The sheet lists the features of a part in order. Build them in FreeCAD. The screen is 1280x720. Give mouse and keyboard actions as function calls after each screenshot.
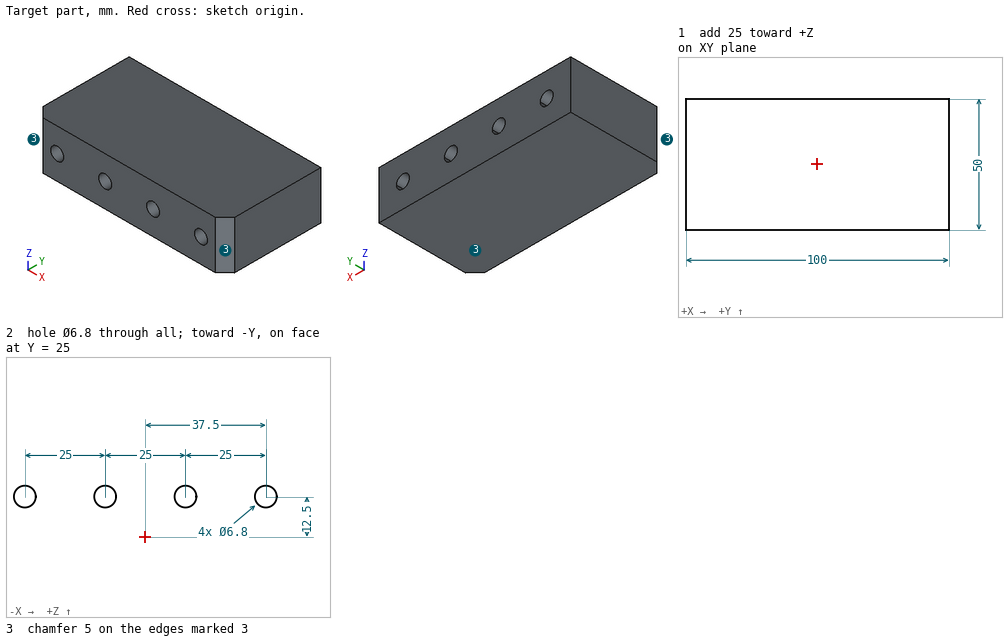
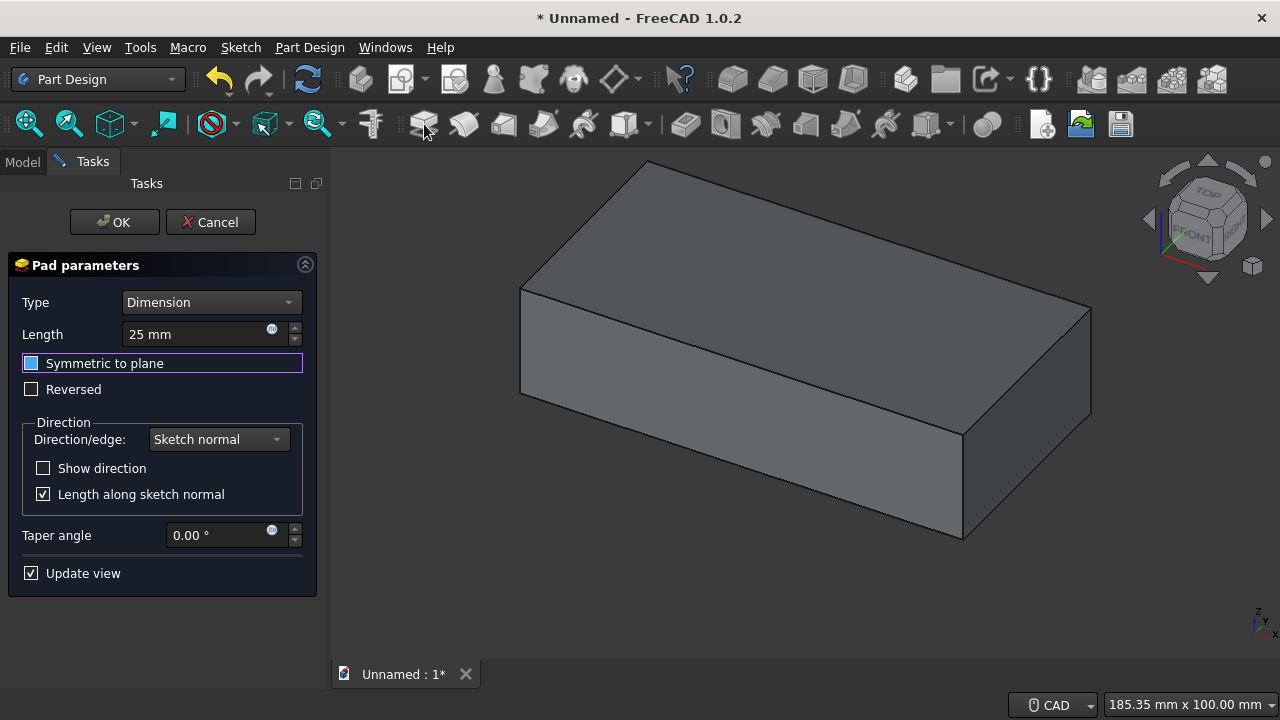
click(115, 222)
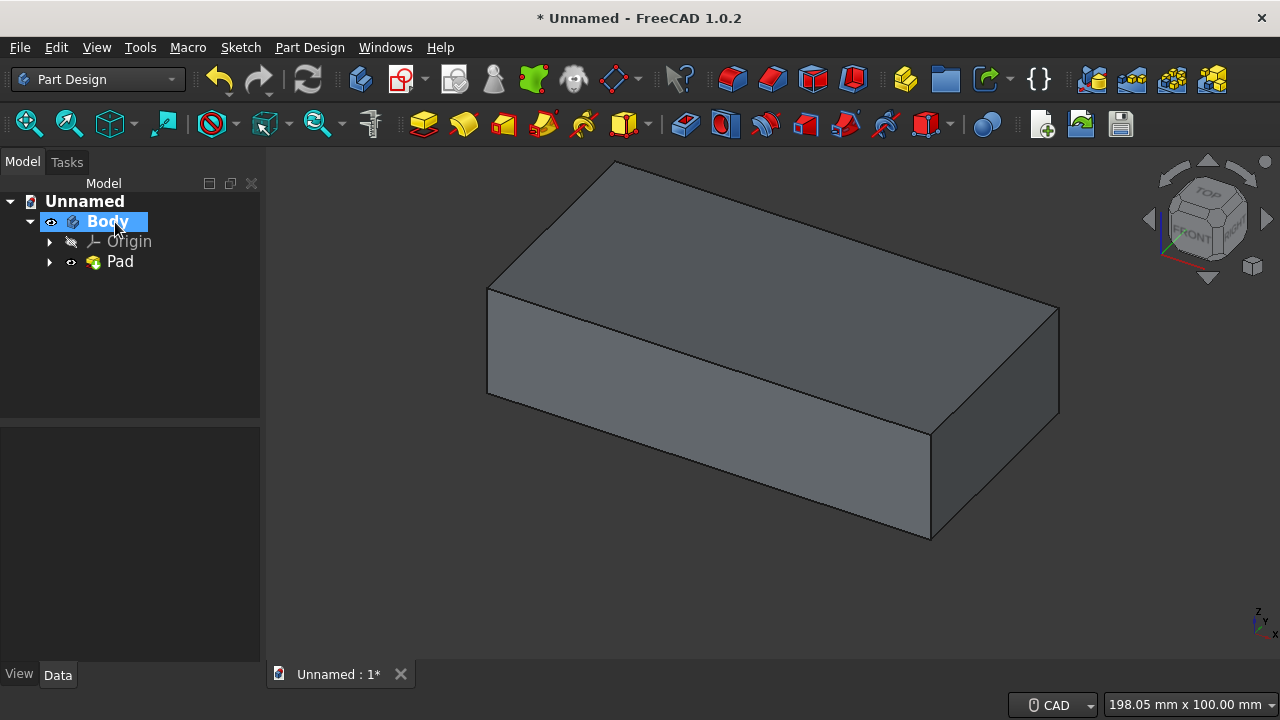
key(4)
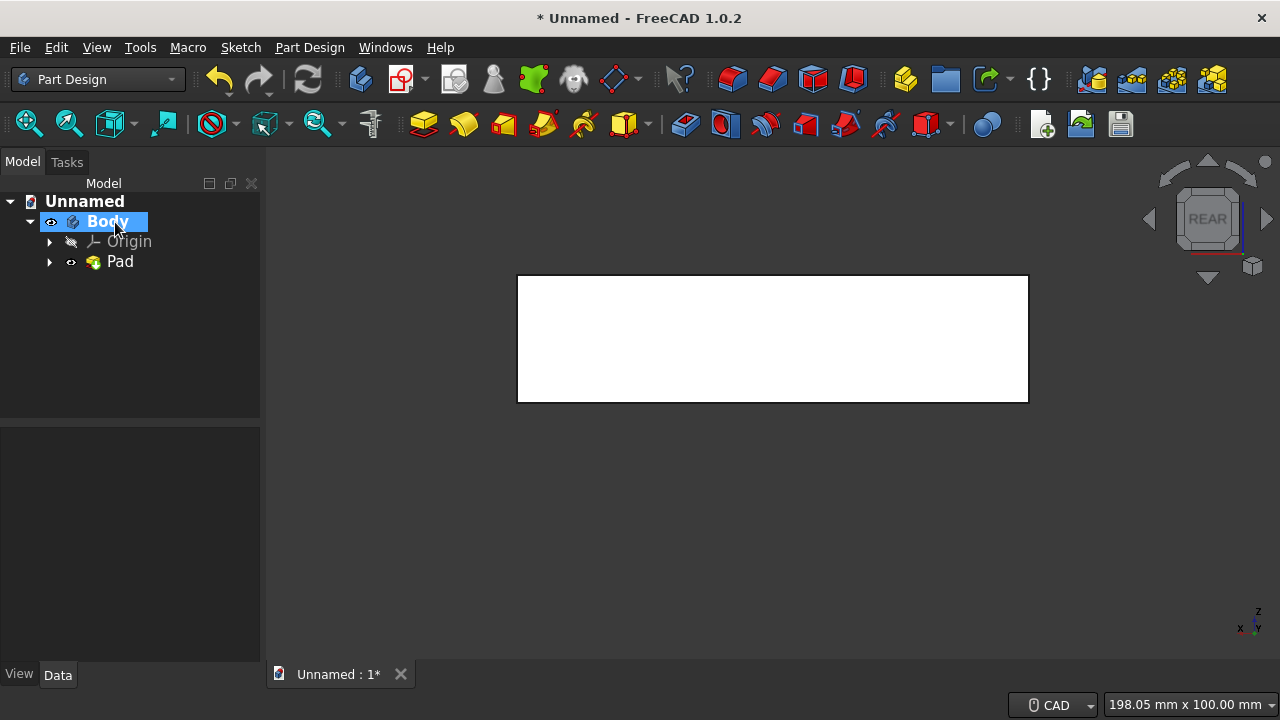
click(627, 338)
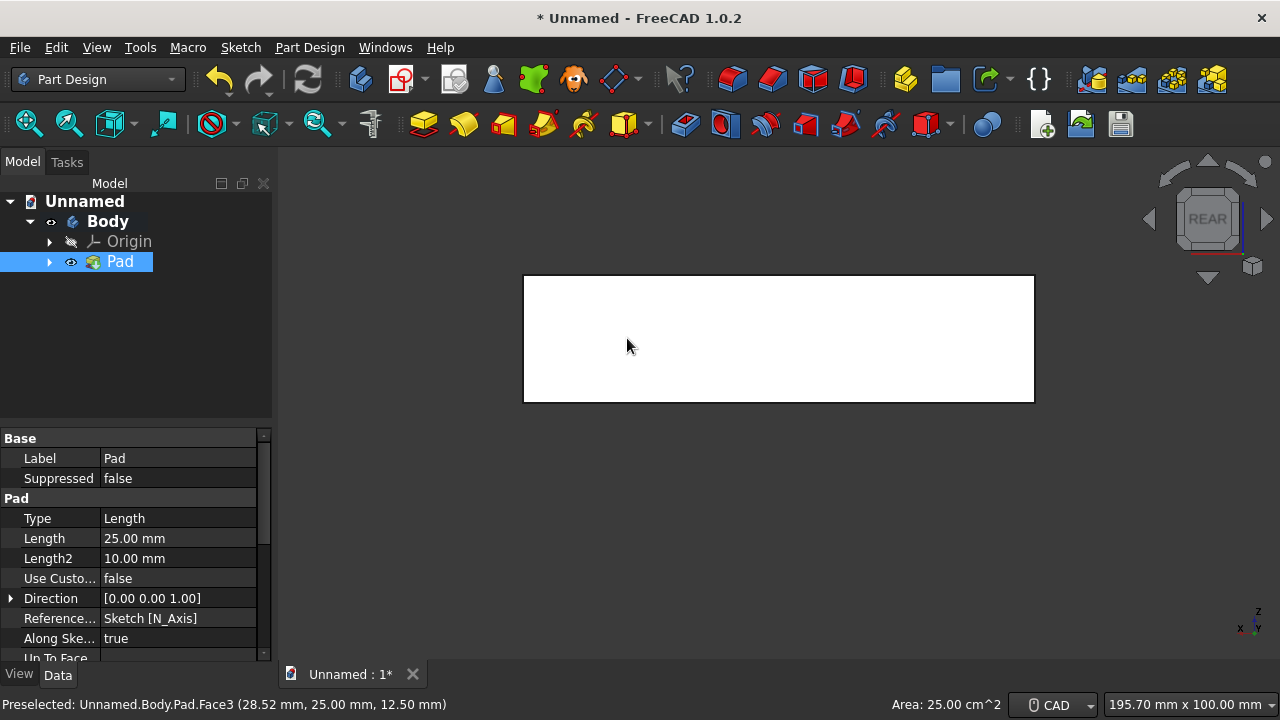
click(402, 80)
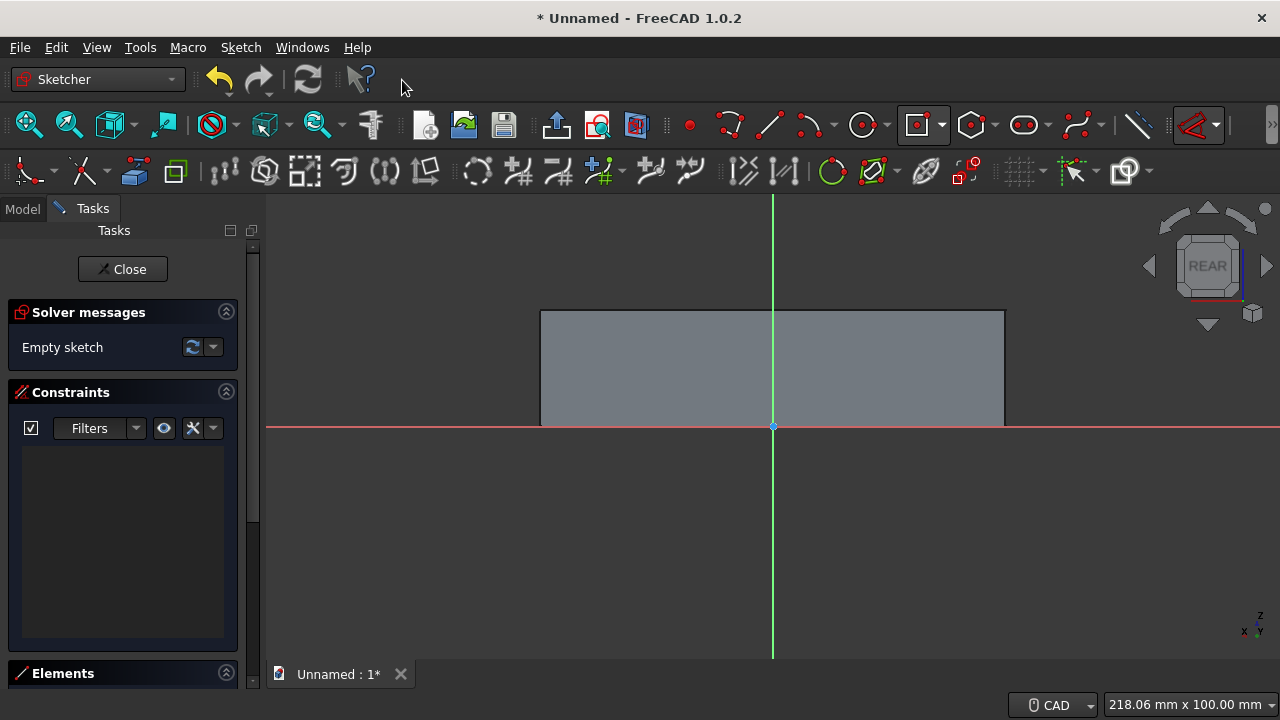
scroll(912, 314, up, 2)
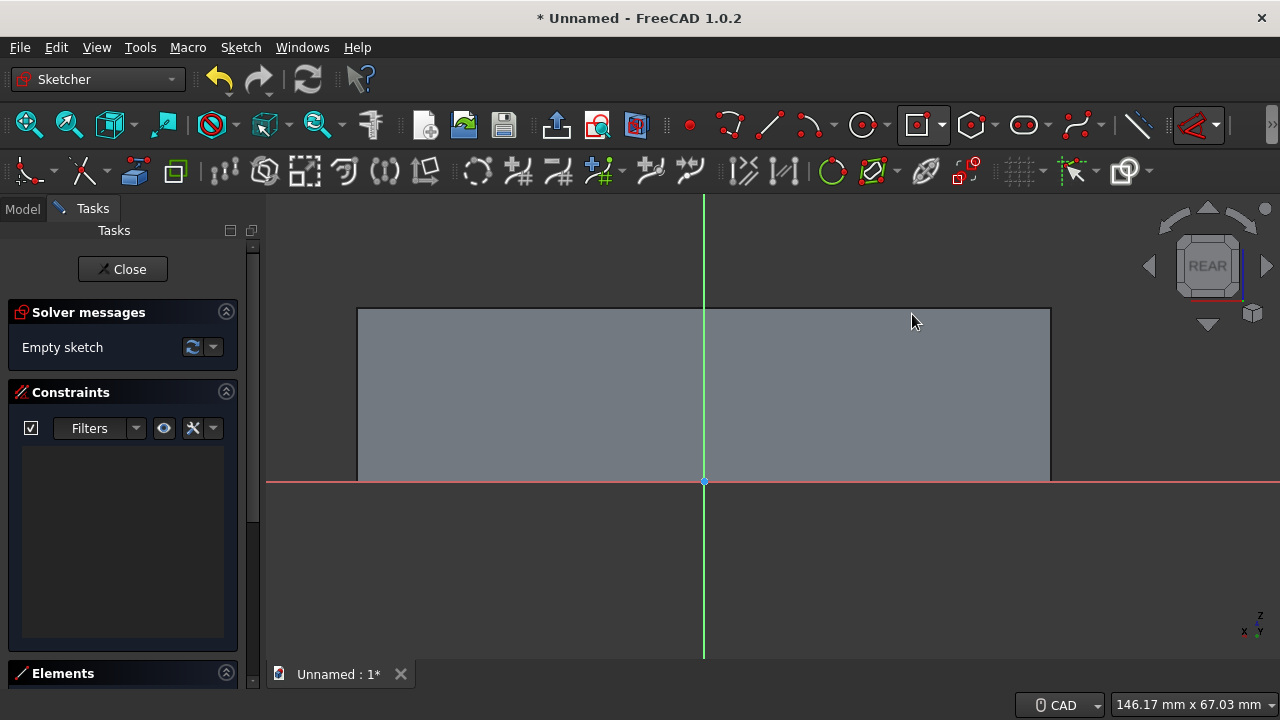
click(864, 126)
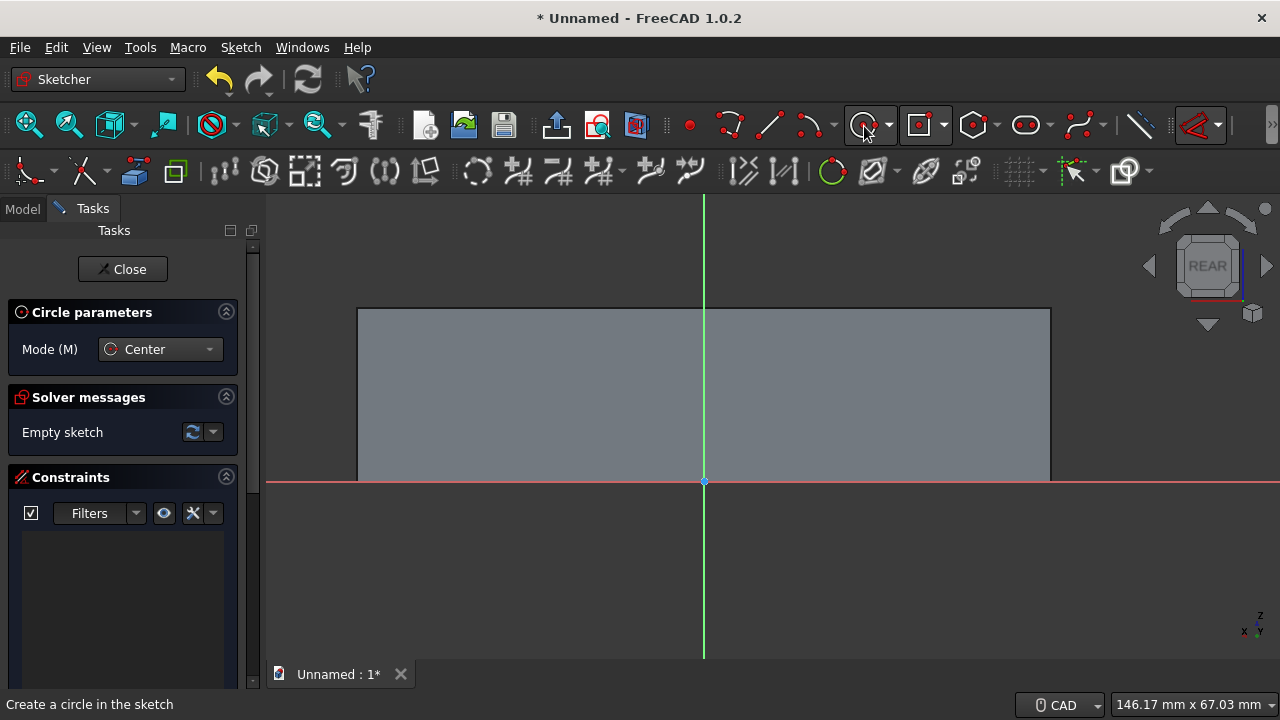
click(964, 395)
move(981, 378)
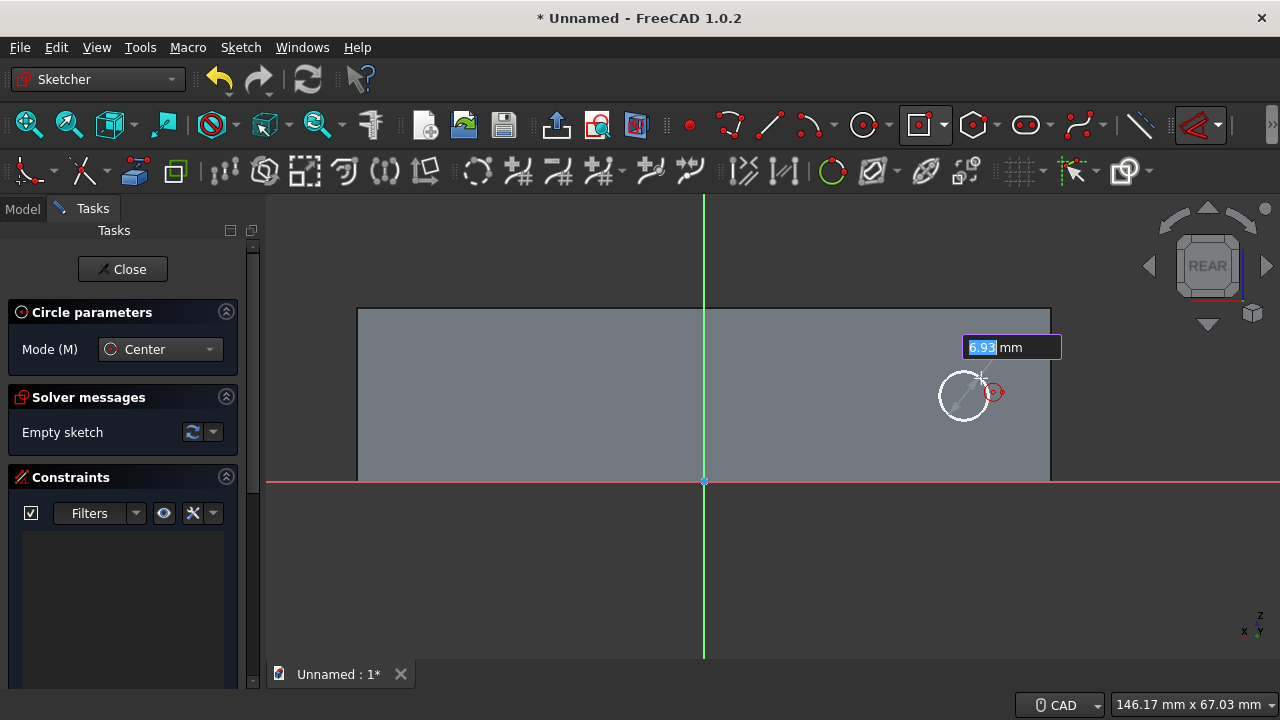
text(6.8)
key(Return)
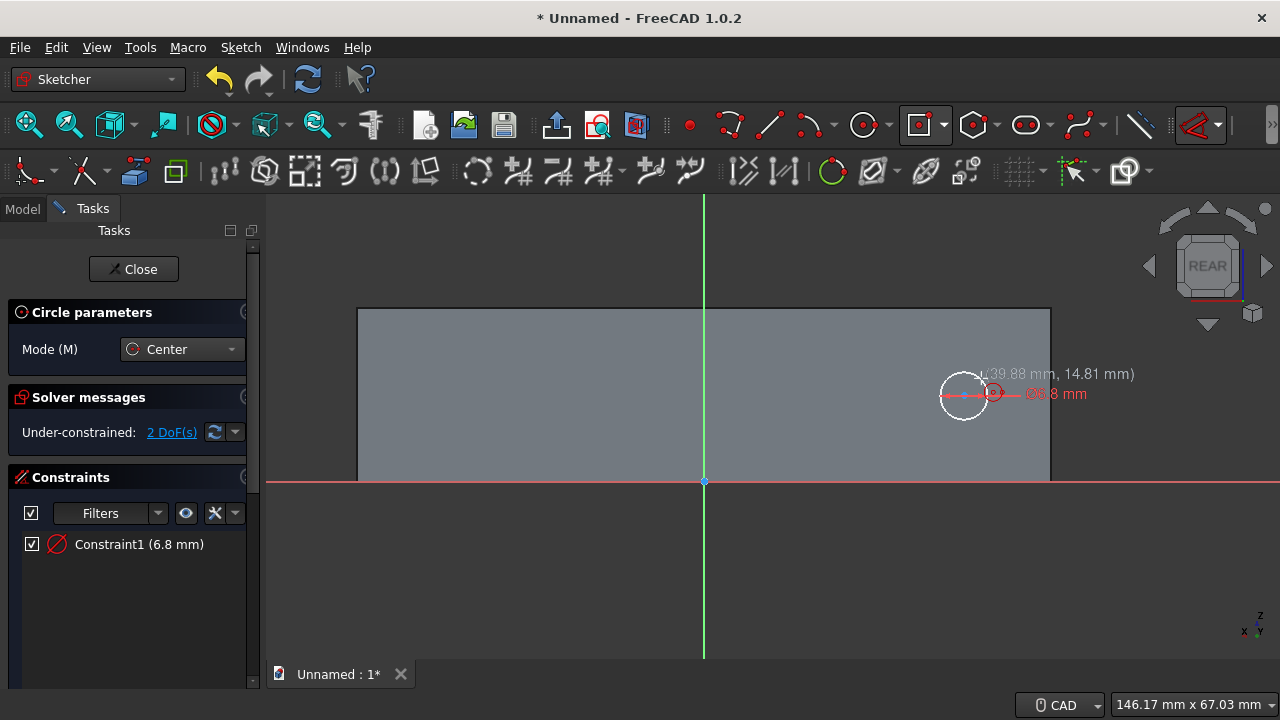
click(791, 395)
move(808, 378)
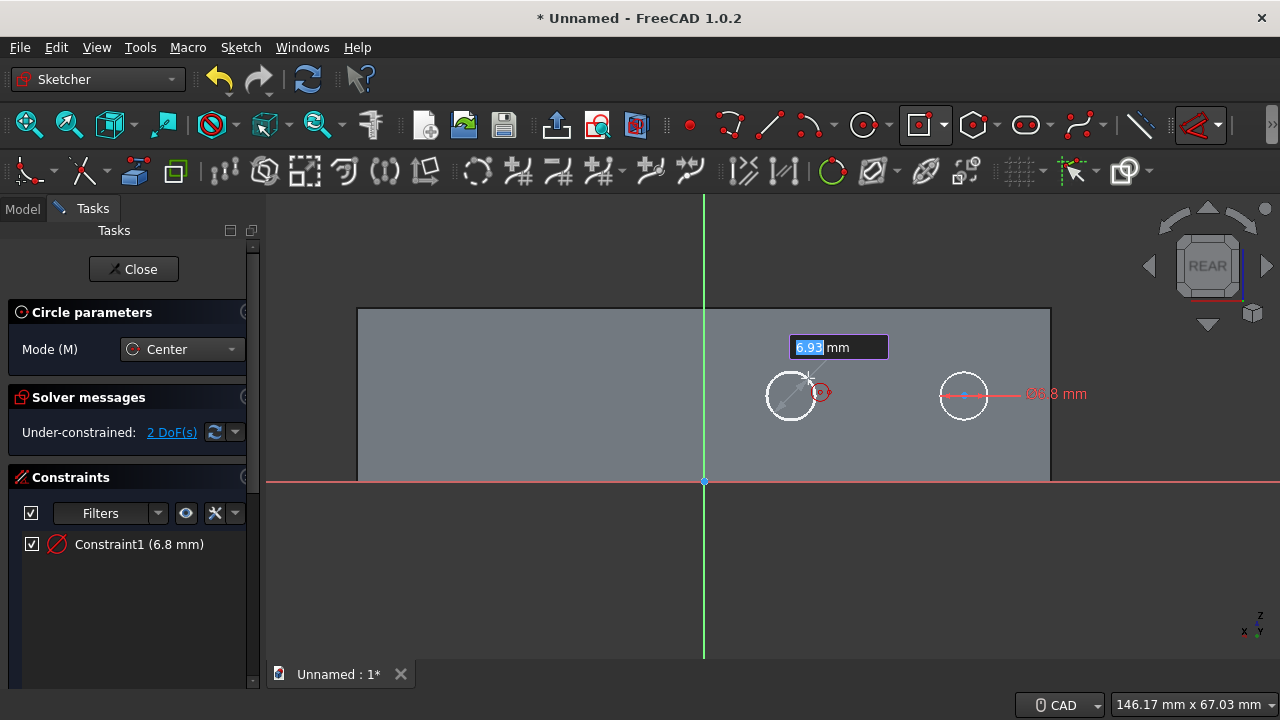
text(6.8)
key(Return)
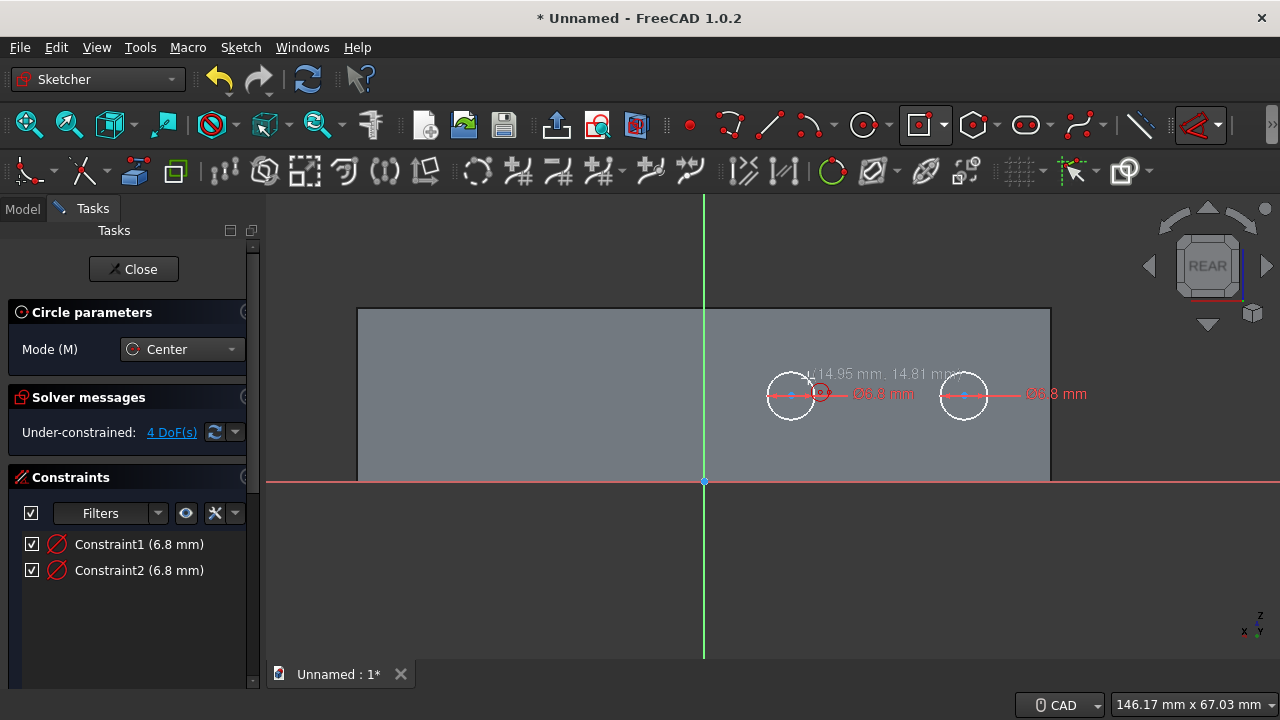
click(618, 395)
move(634, 378)